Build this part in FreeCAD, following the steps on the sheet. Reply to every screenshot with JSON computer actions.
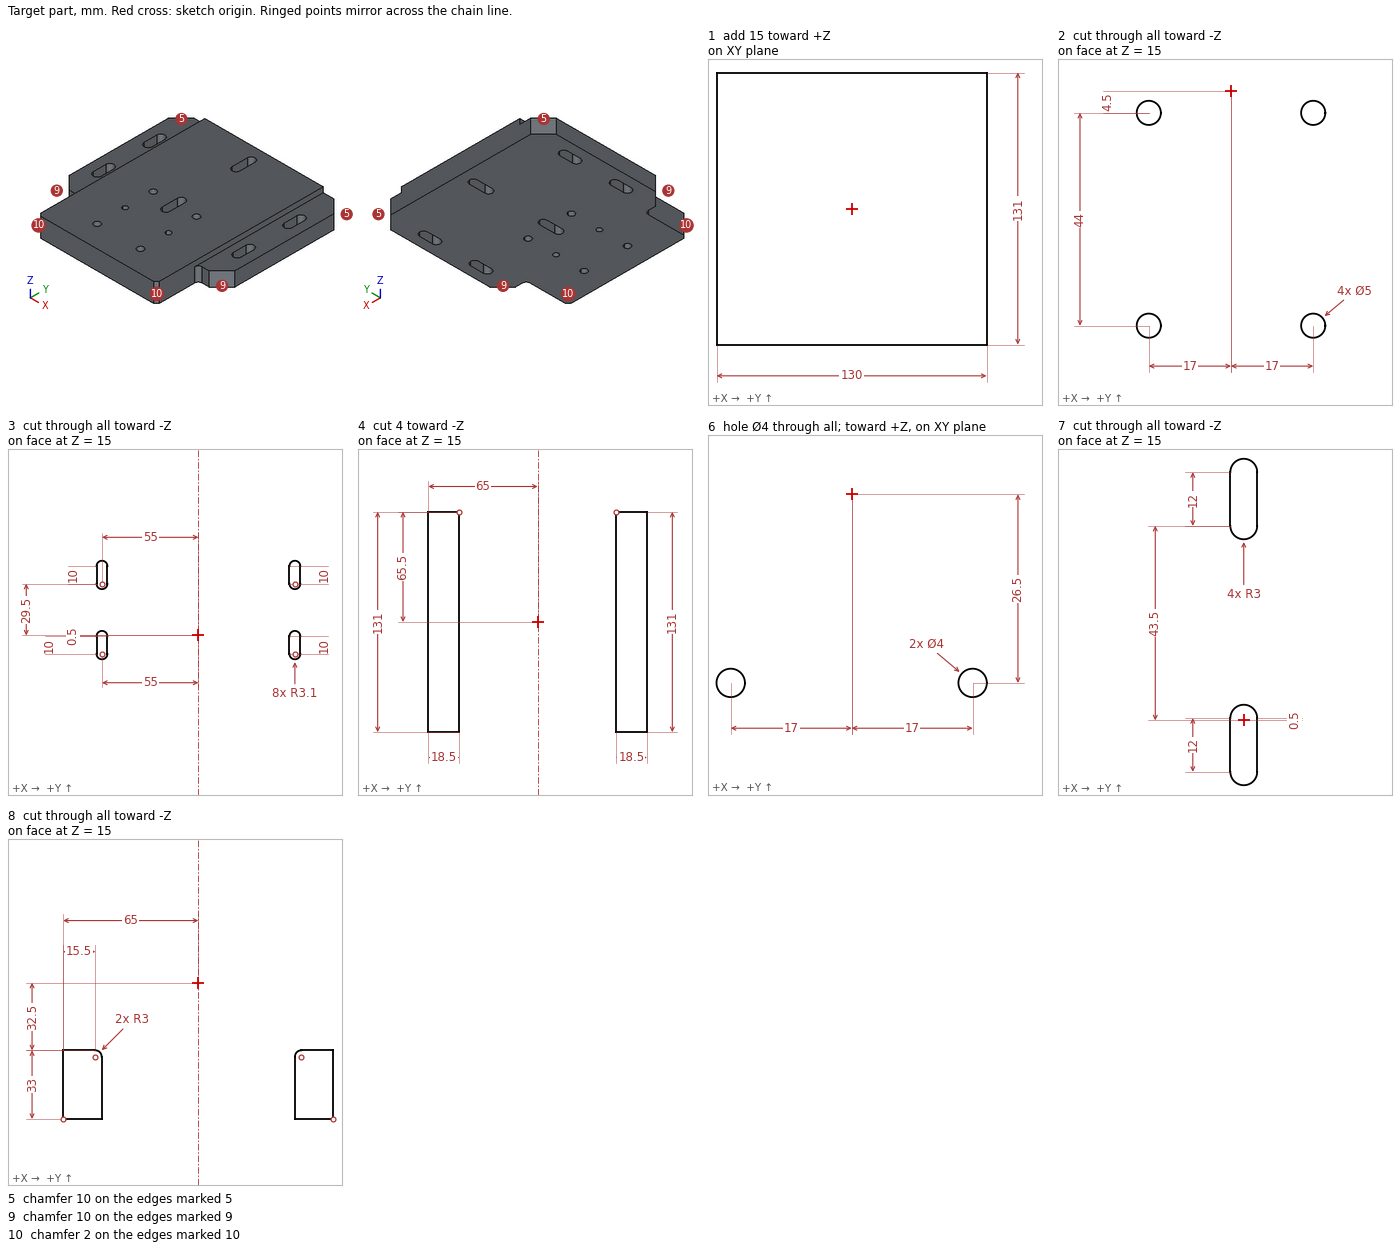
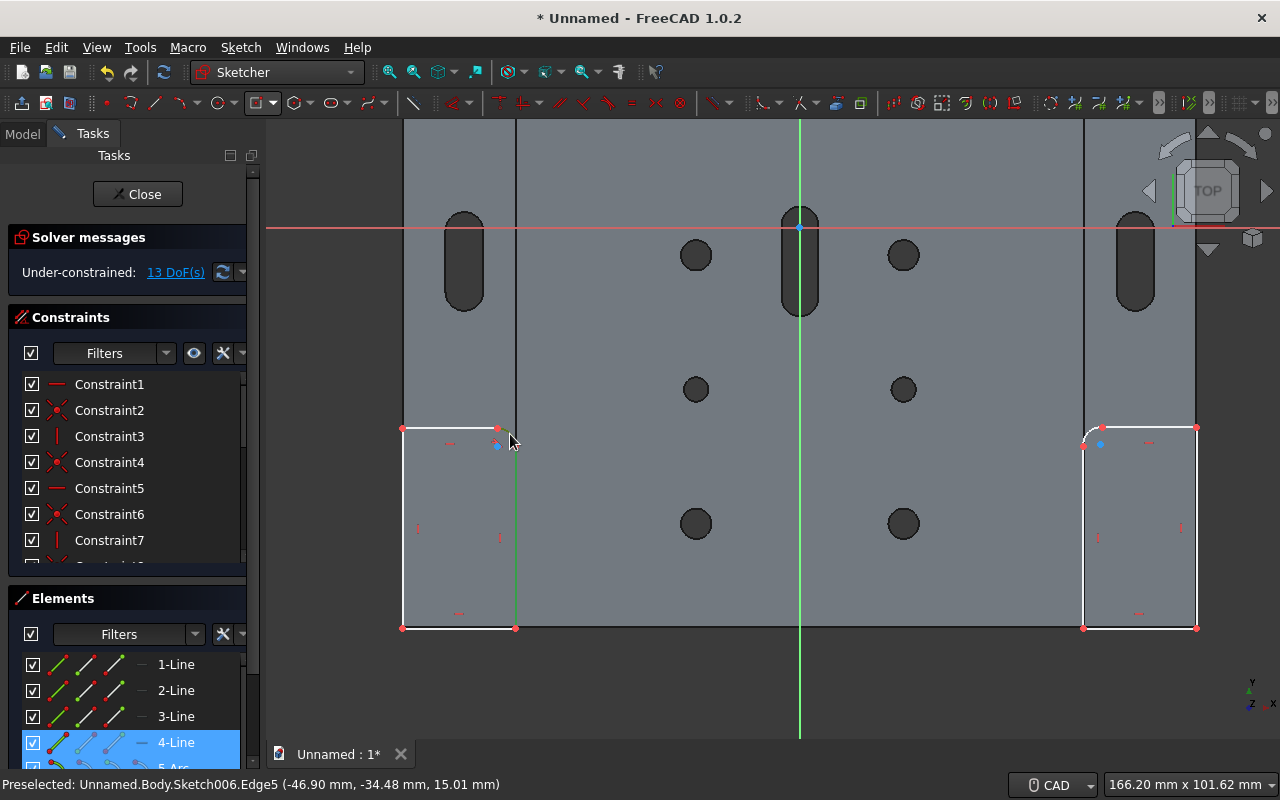
{"action": "key", "text": "t"}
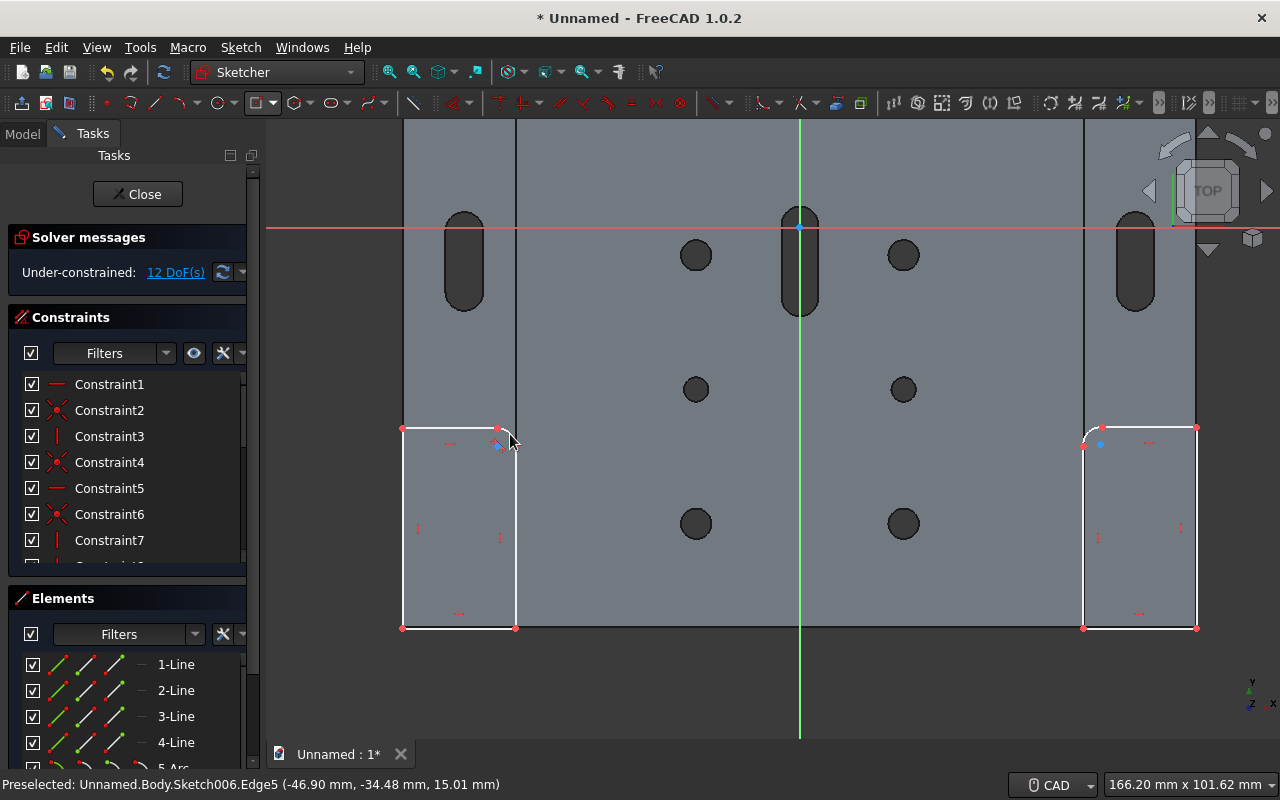
{"action": "left_click", "coordinate": [1083, 501]}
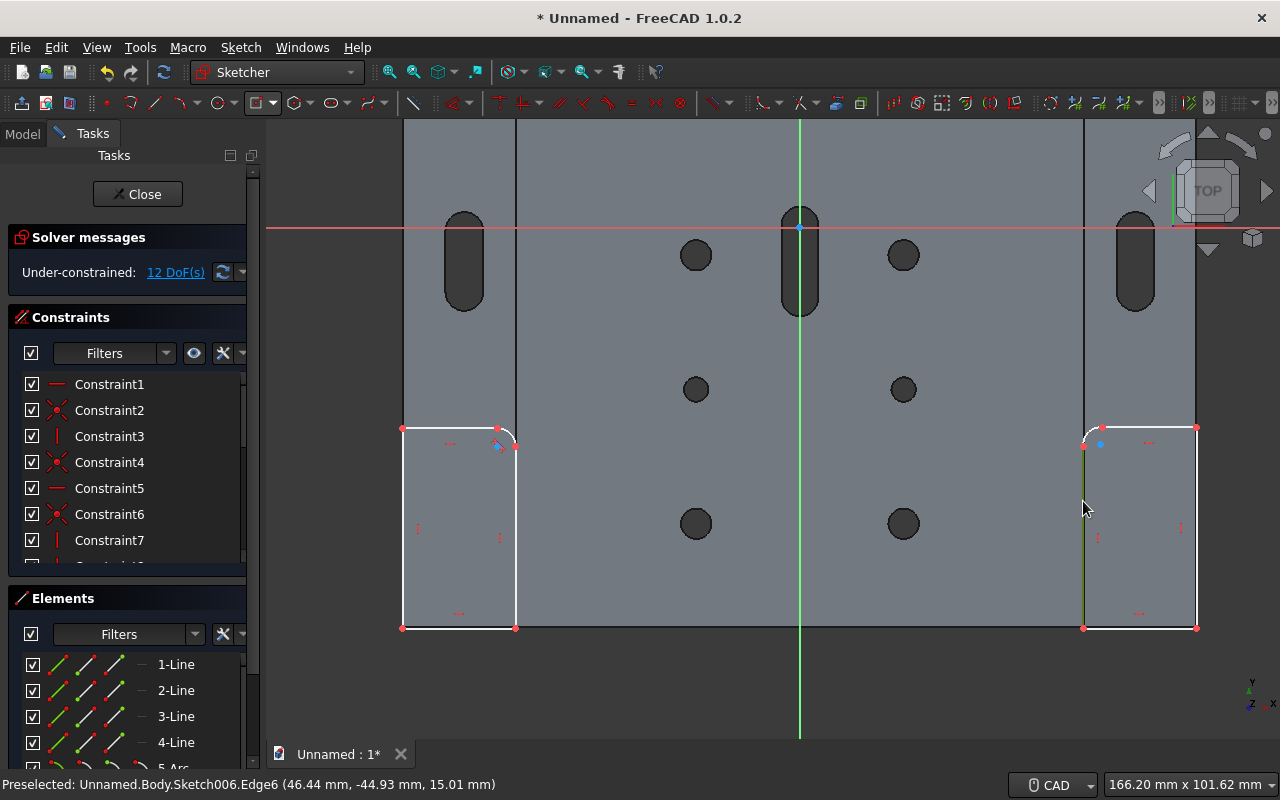
{"action": "scroll", "coordinate": [1093, 429], "scroll_direction": "up", "scroll_amount": 2}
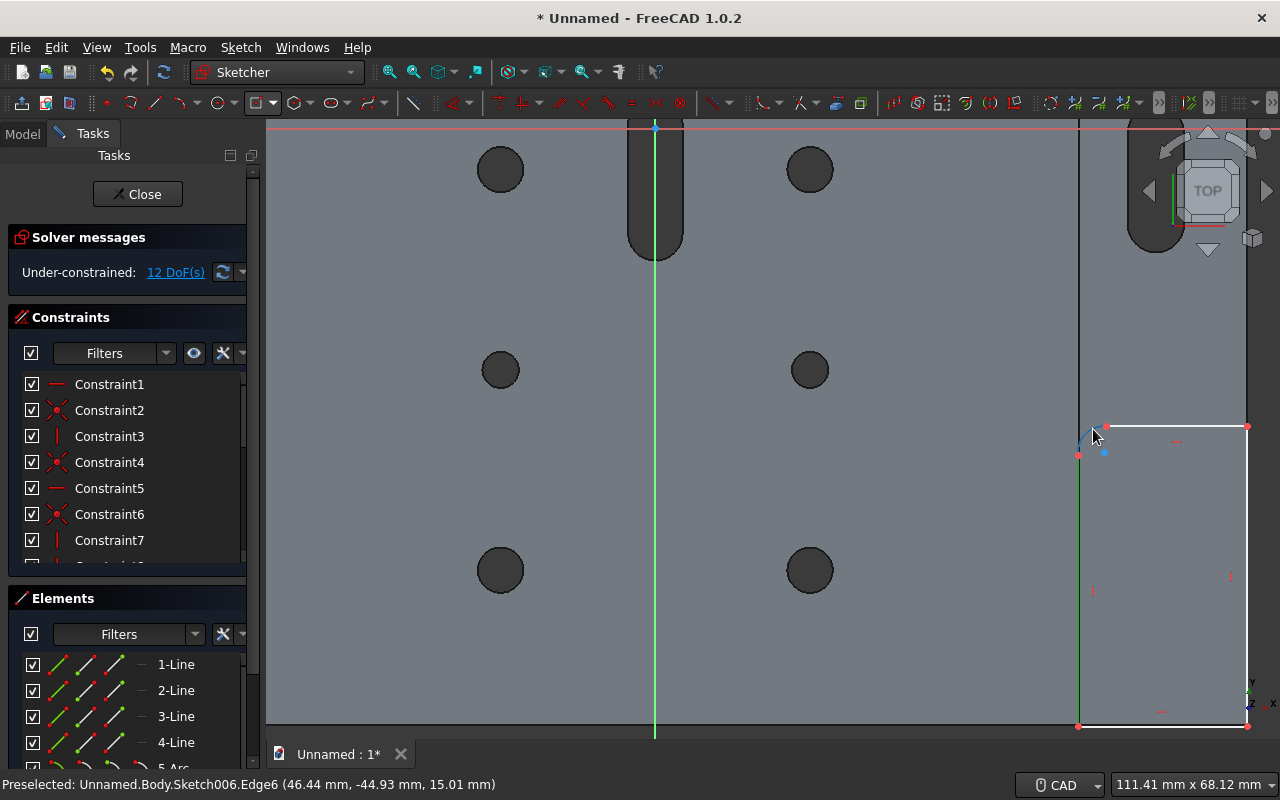
{"action": "left_click", "coordinate": [1093, 429]}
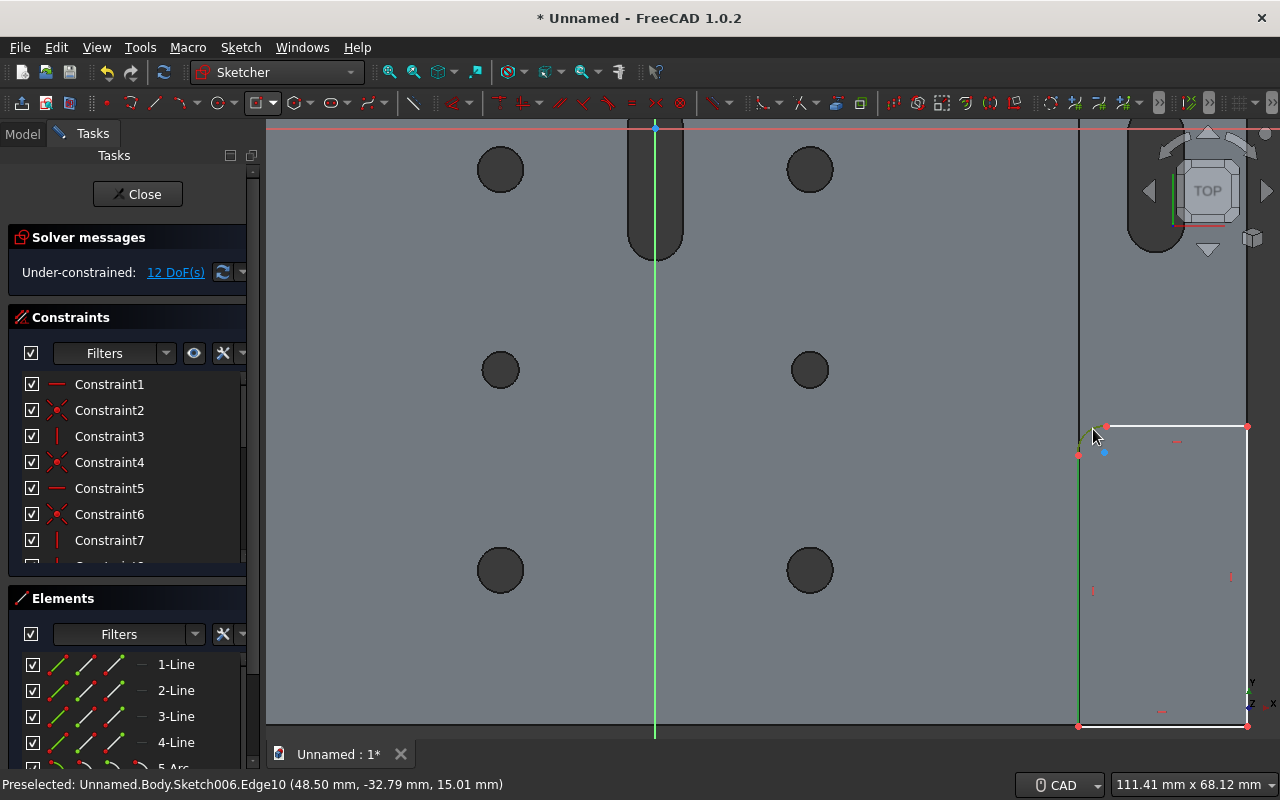
{"action": "key", "text": "t"}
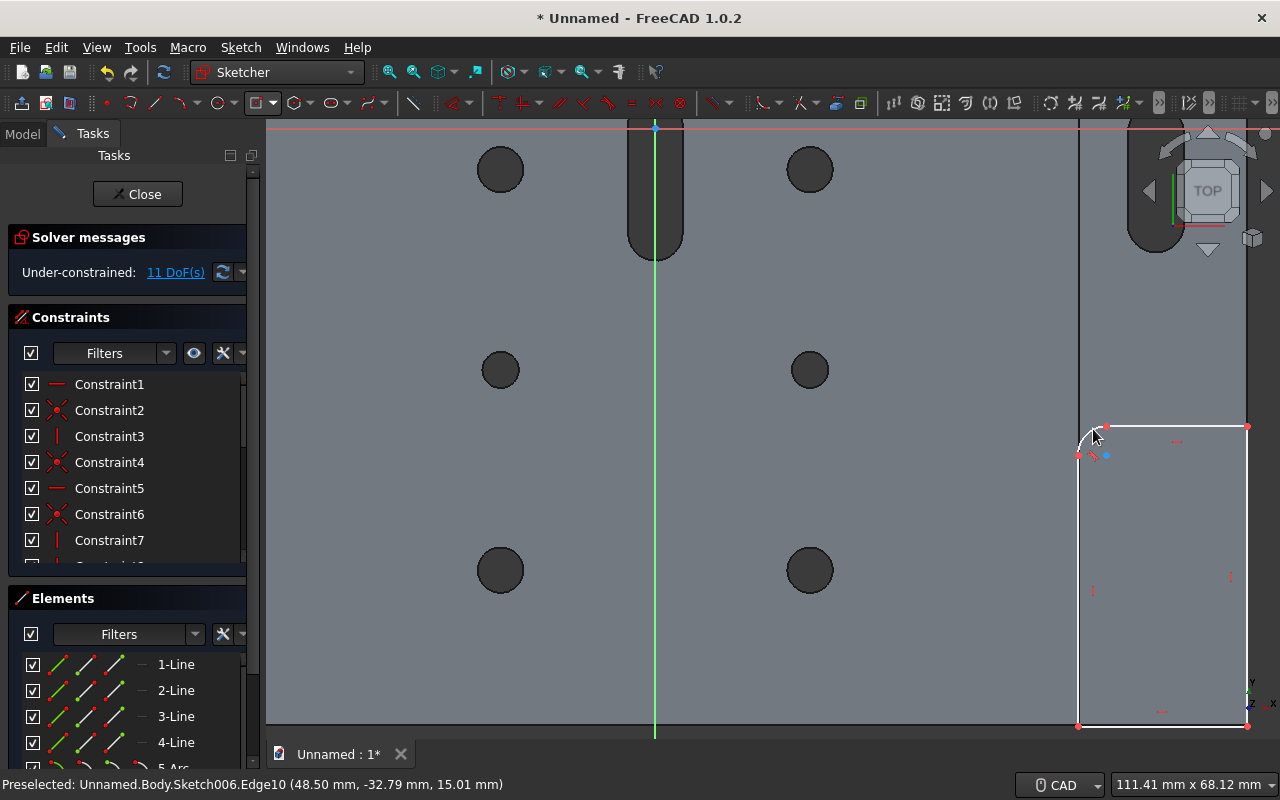
{"action": "scroll", "coordinate": [745, 431], "scroll_direction": "down", "scroll_amount": 4}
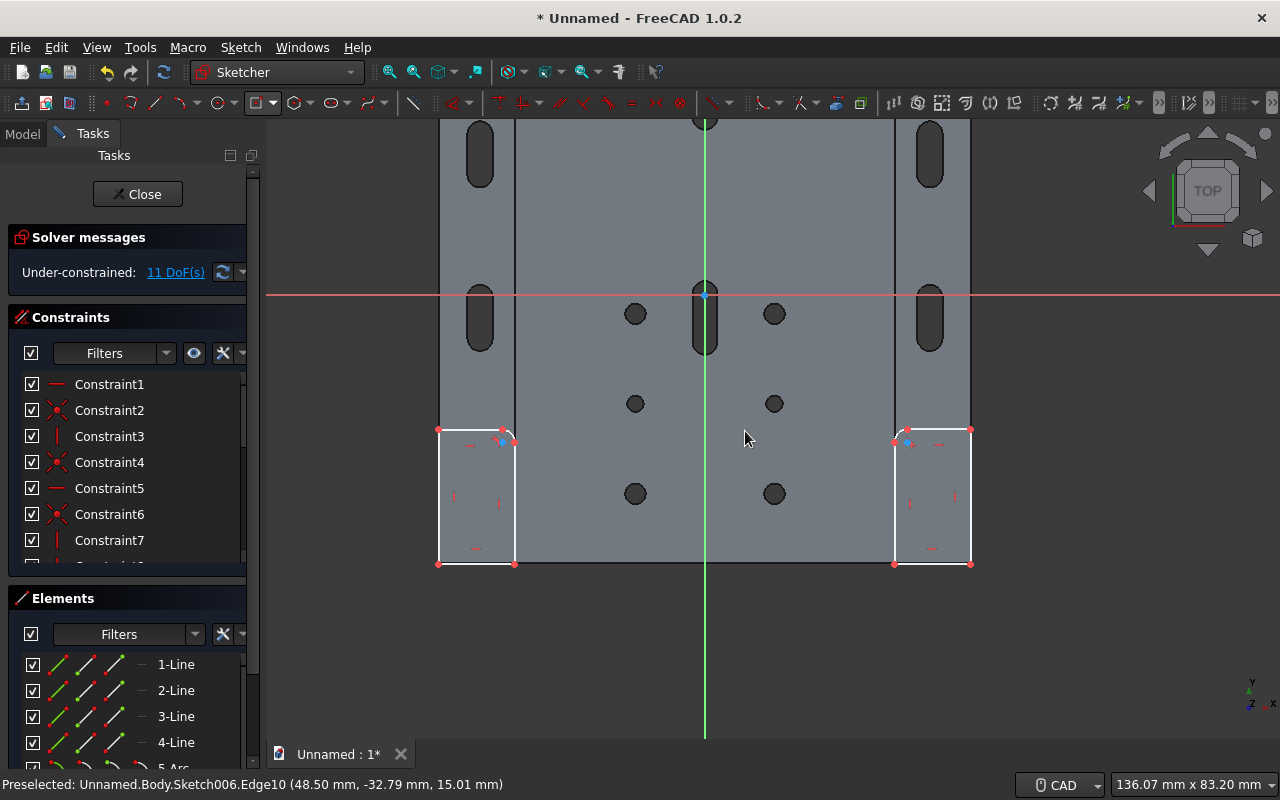
{"action": "left_click", "coordinate": [952, 429]}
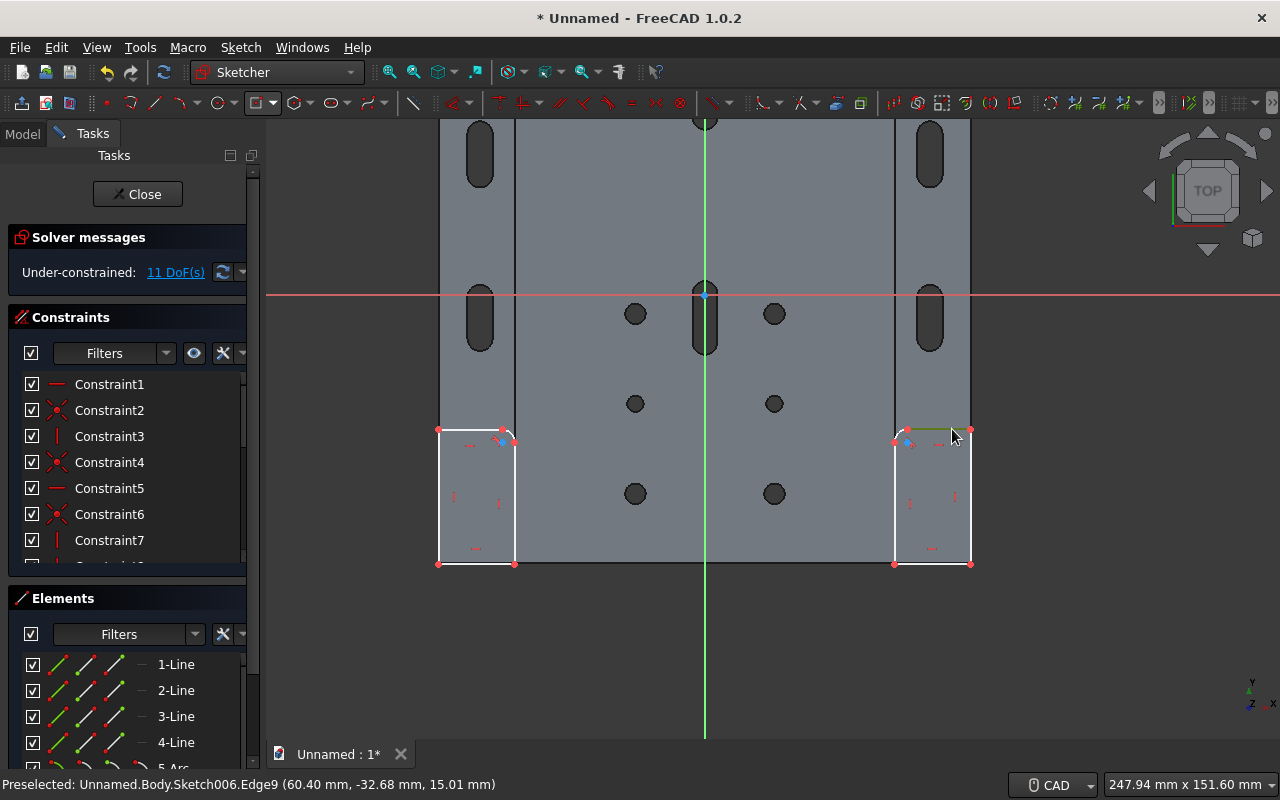
{"action": "scroll", "coordinate": [899, 433], "scroll_direction": "up", "scroll_amount": 2}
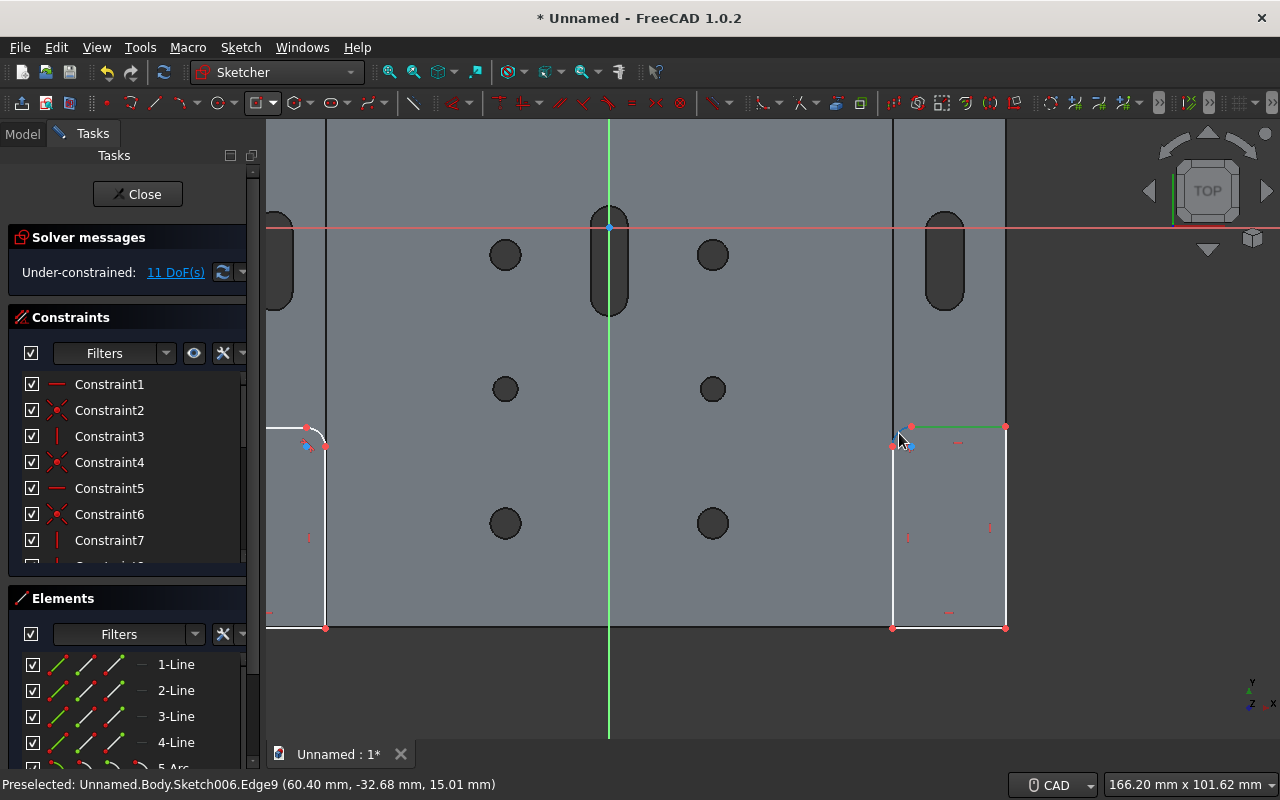
{"action": "left_click", "coordinate": [898, 433]}